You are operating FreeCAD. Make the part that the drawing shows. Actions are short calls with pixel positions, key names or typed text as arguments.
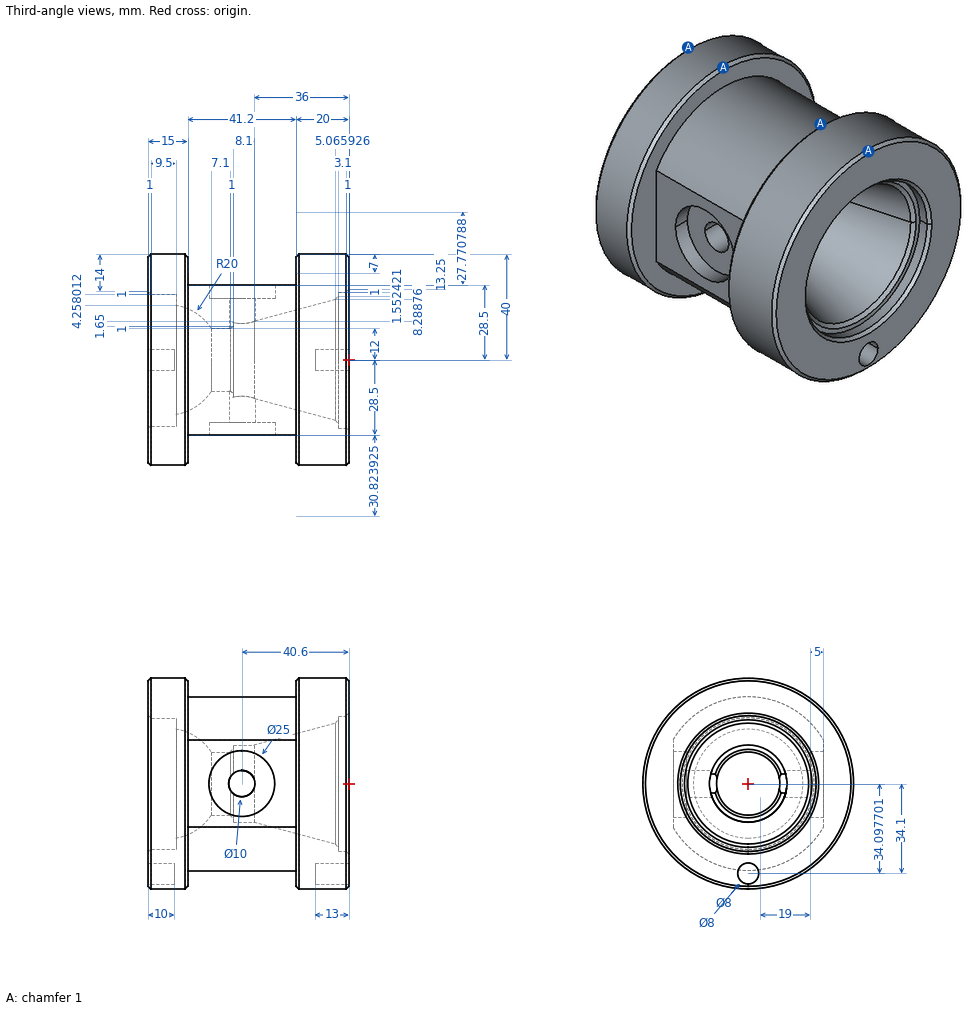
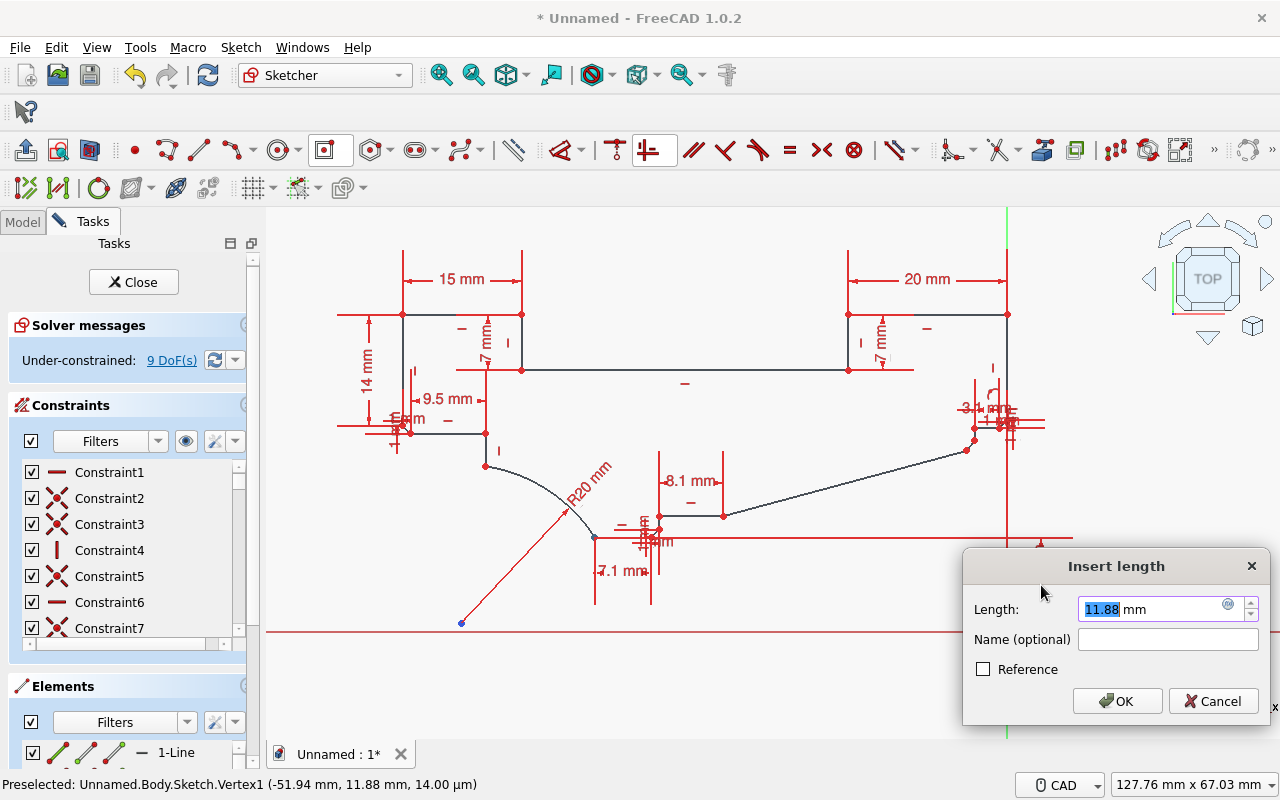
text(12)
key(Return)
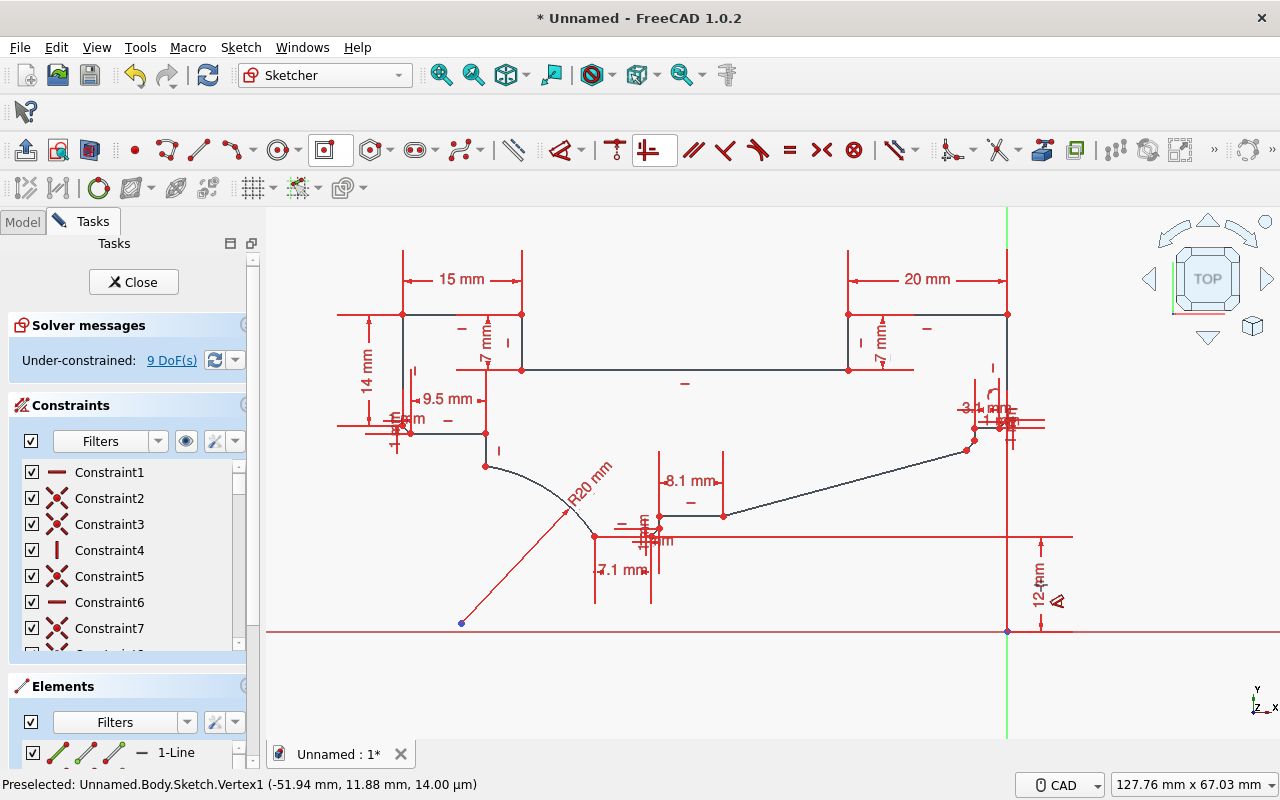
click(723, 516)
click(865, 666)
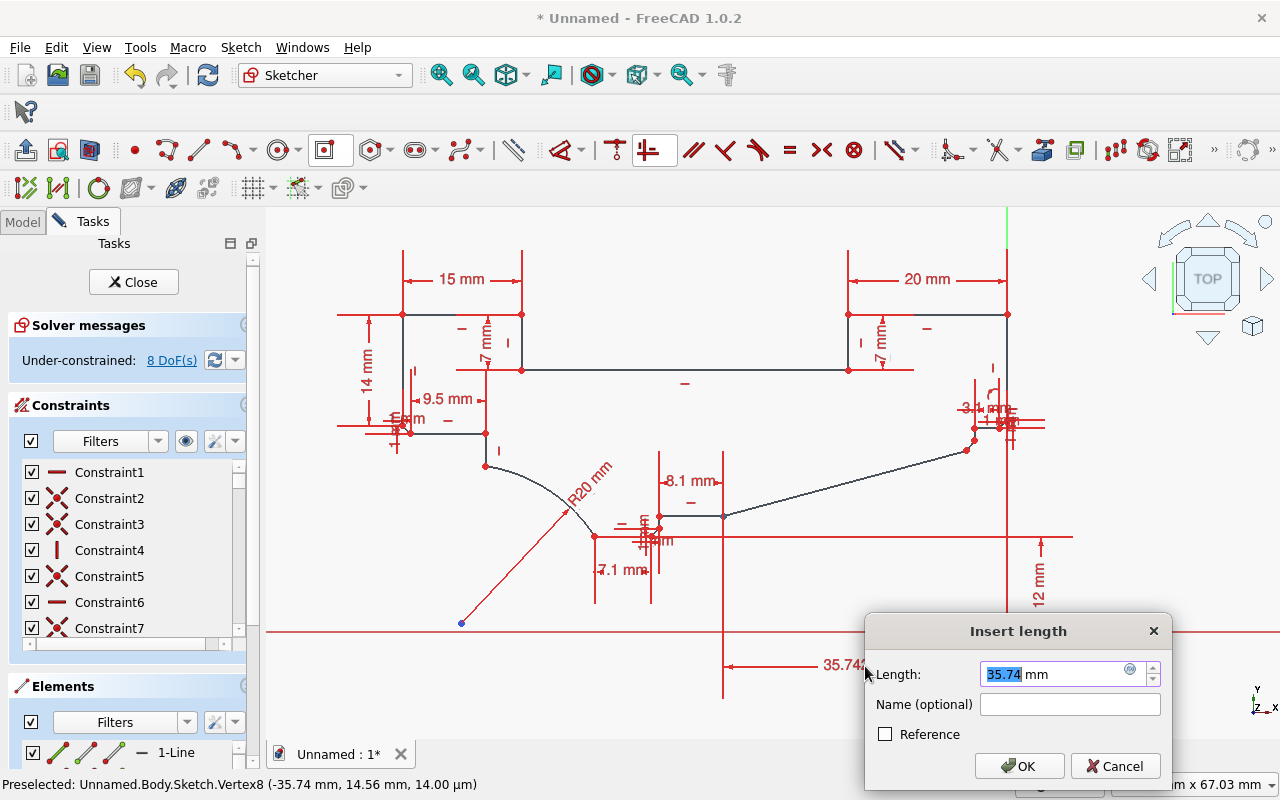
text(36)
key(Return)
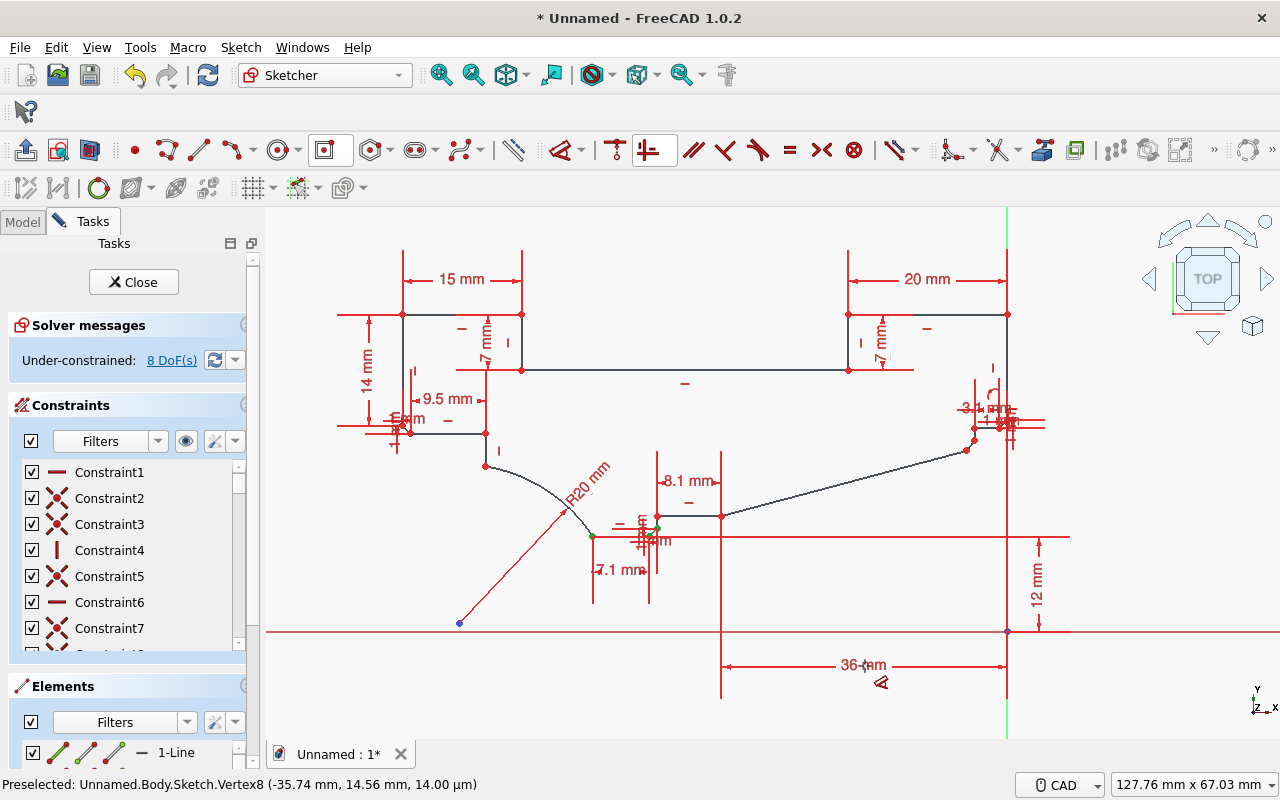
click(1007, 315)
click(1041, 473)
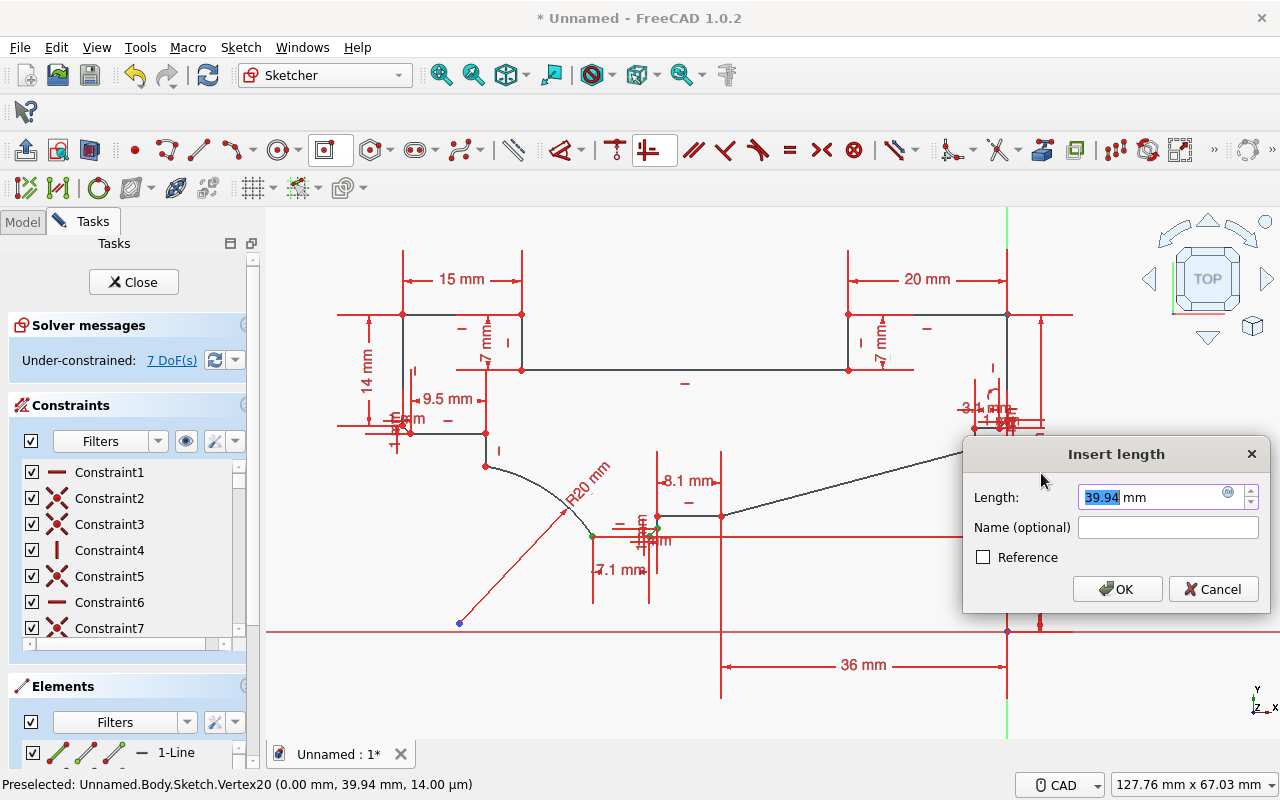
text(40)
key(Return)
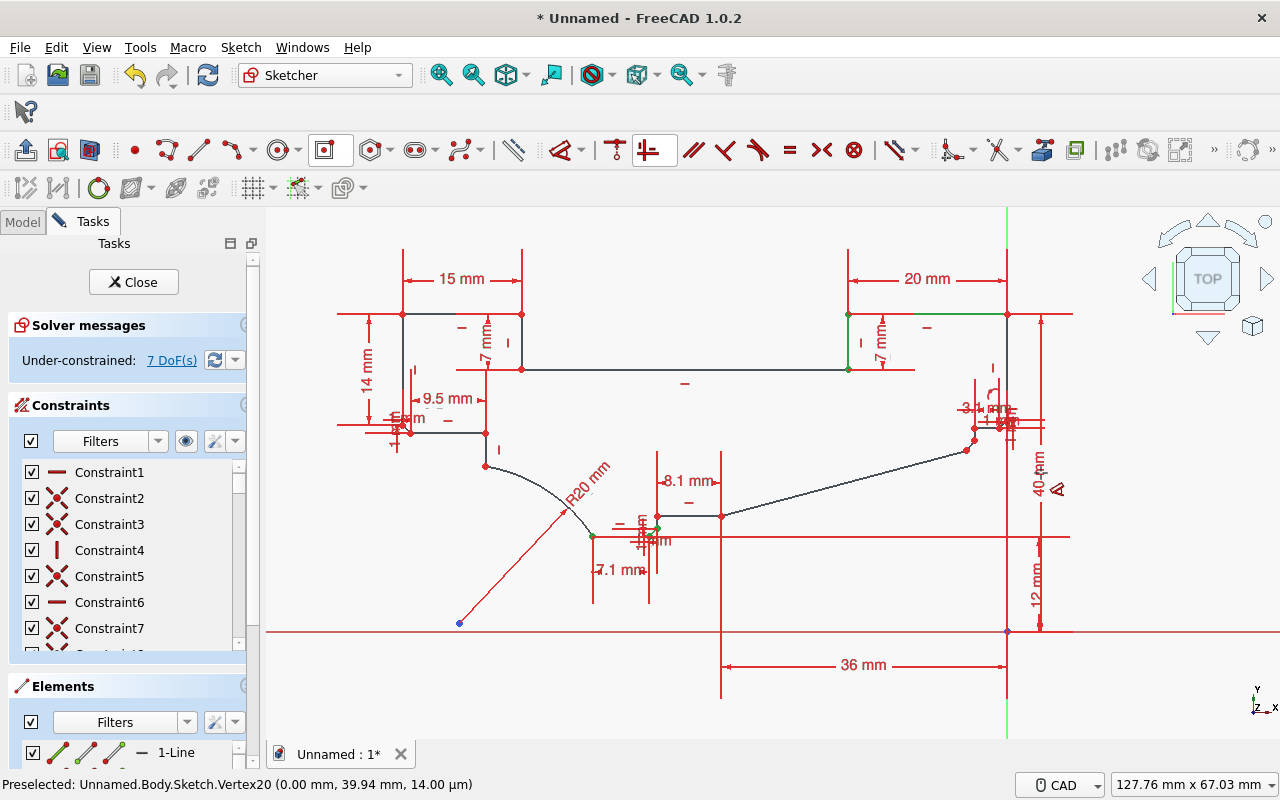
scroll(657, 522, up, 6)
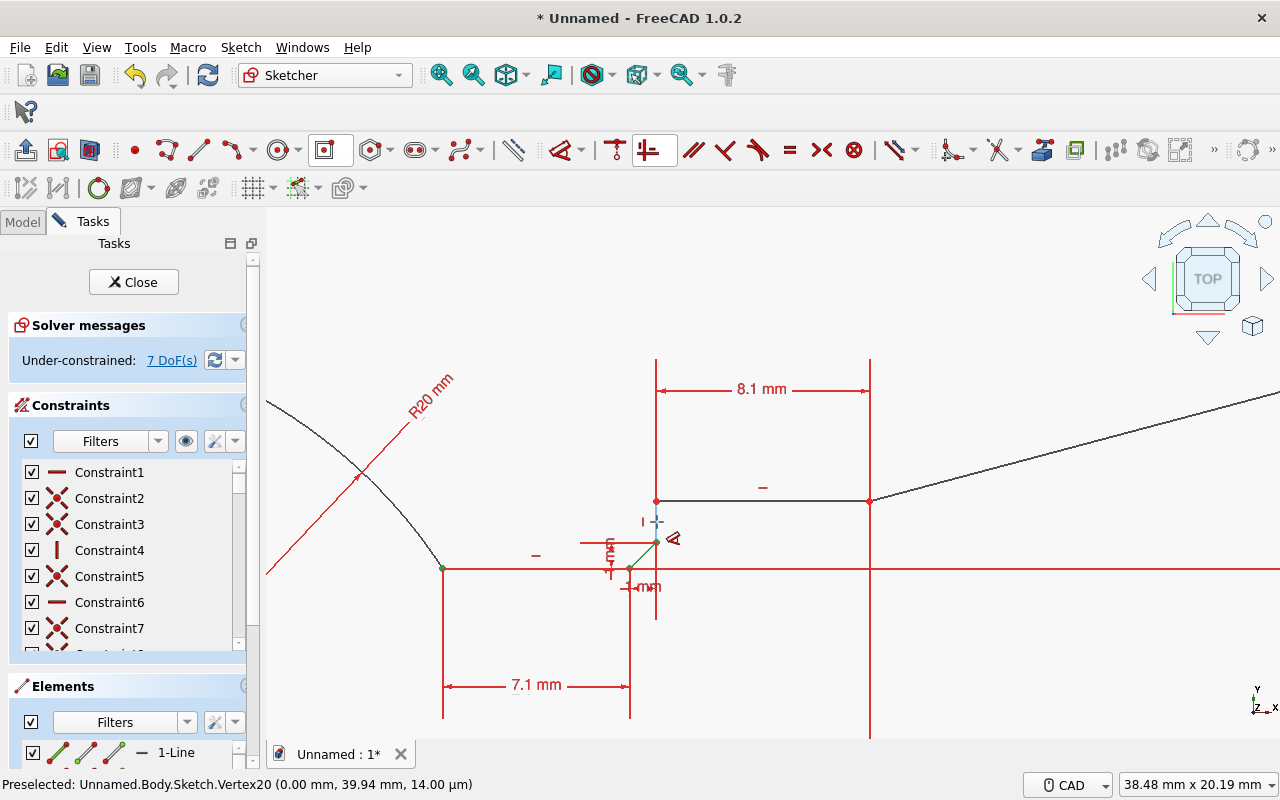
click(656, 522)
click(622, 522)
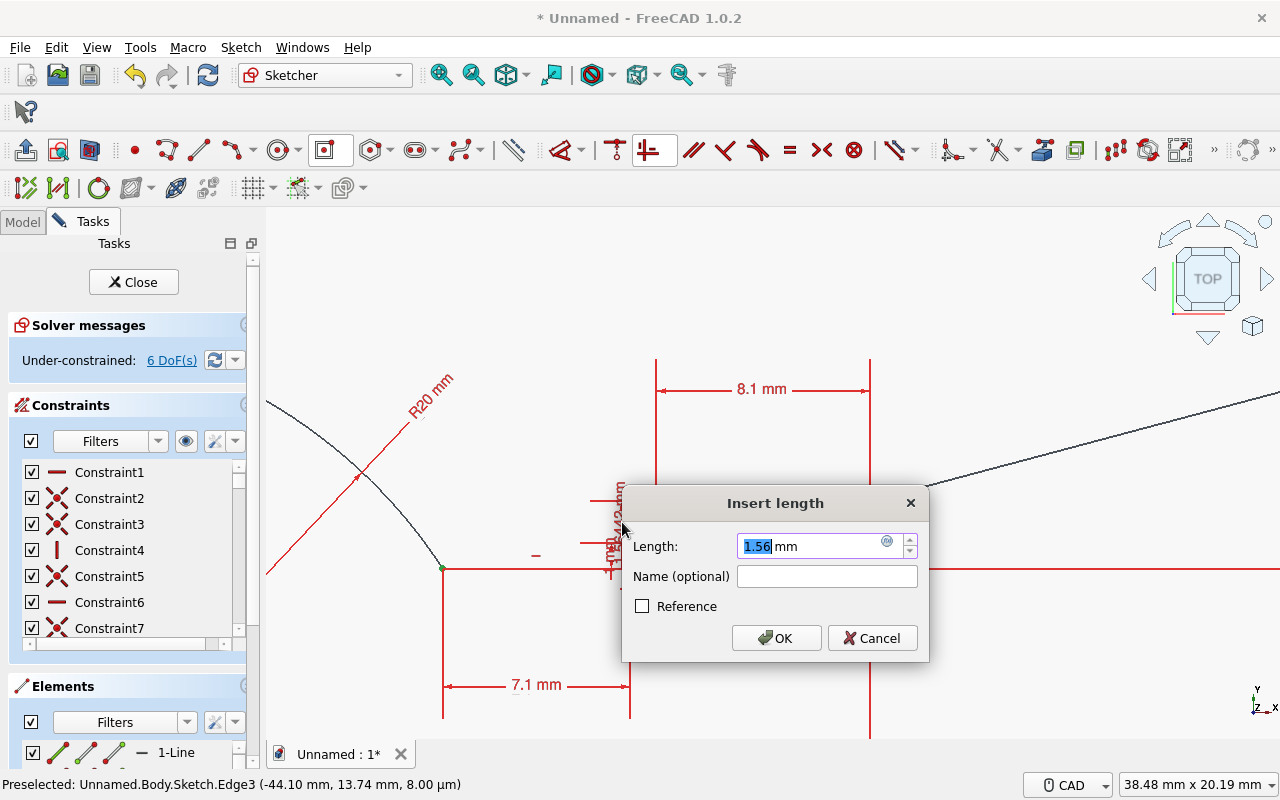
text(1.65)
key(Return)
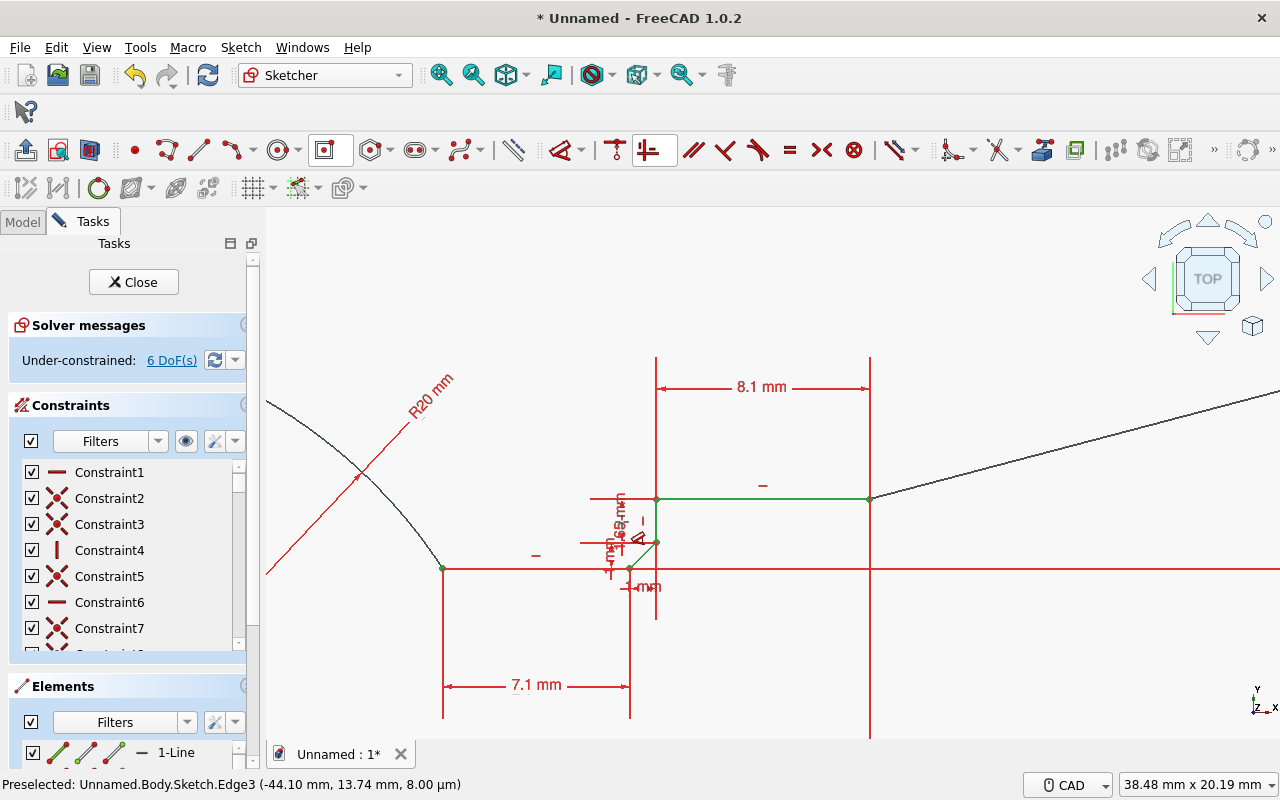
scroll(657, 523, down, 6)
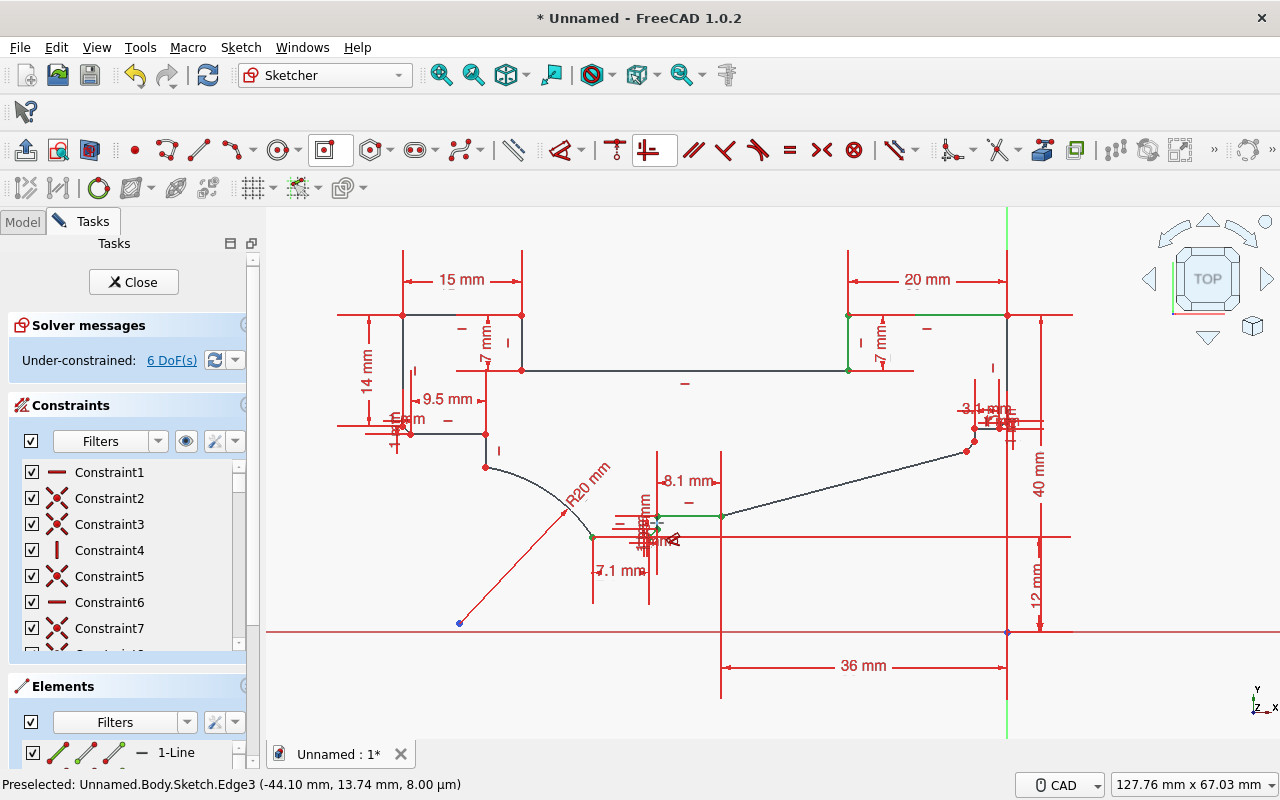
click(750, 371)
click(685, 337)